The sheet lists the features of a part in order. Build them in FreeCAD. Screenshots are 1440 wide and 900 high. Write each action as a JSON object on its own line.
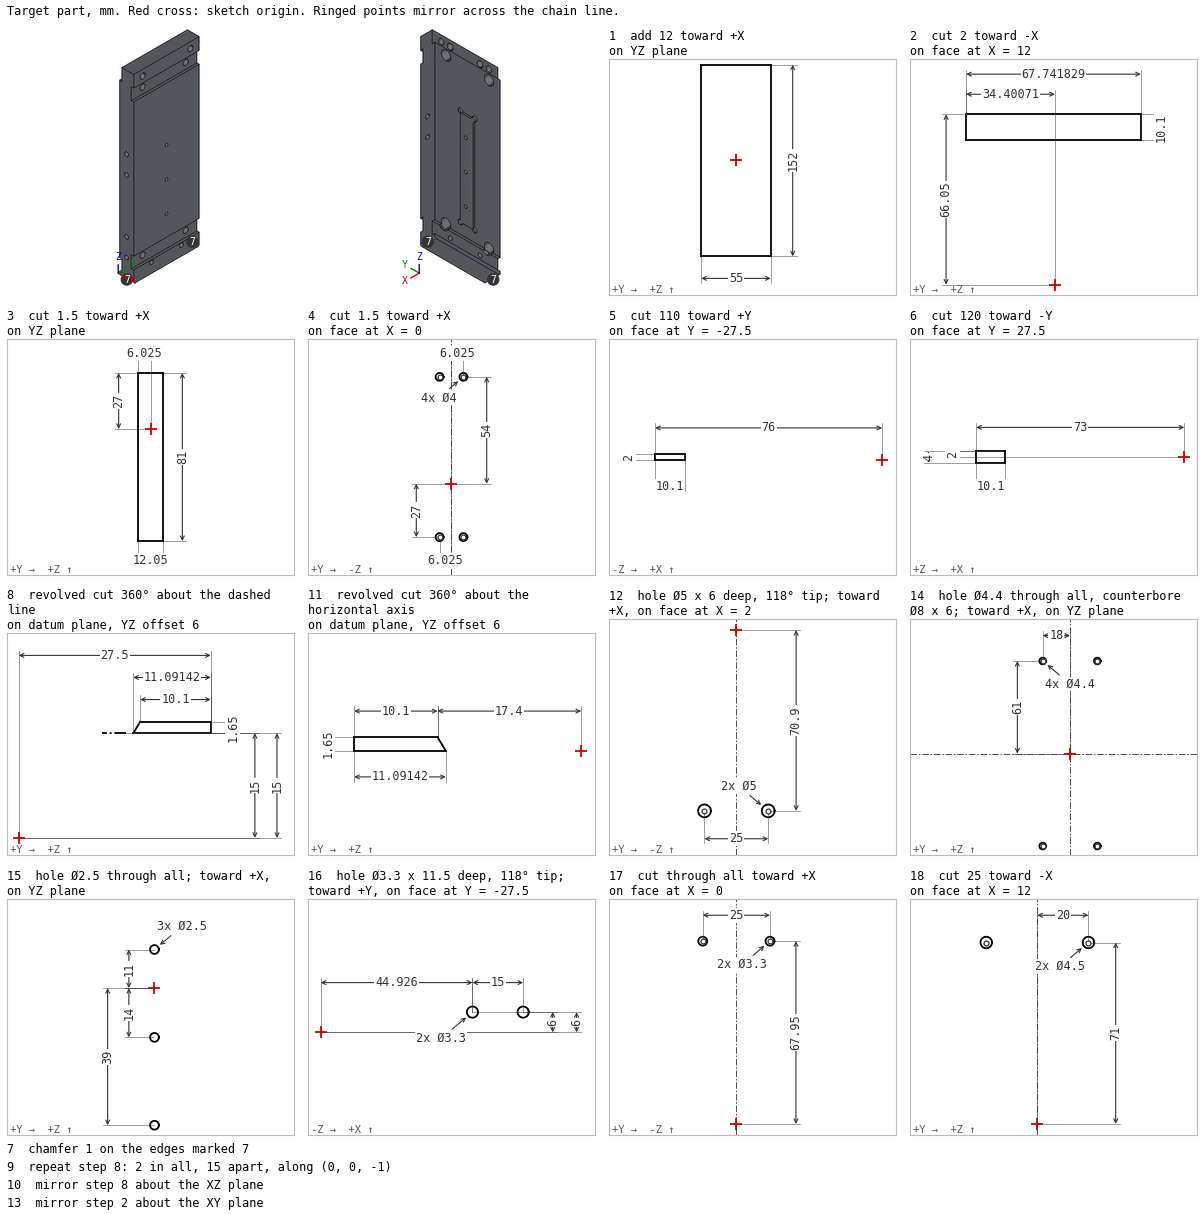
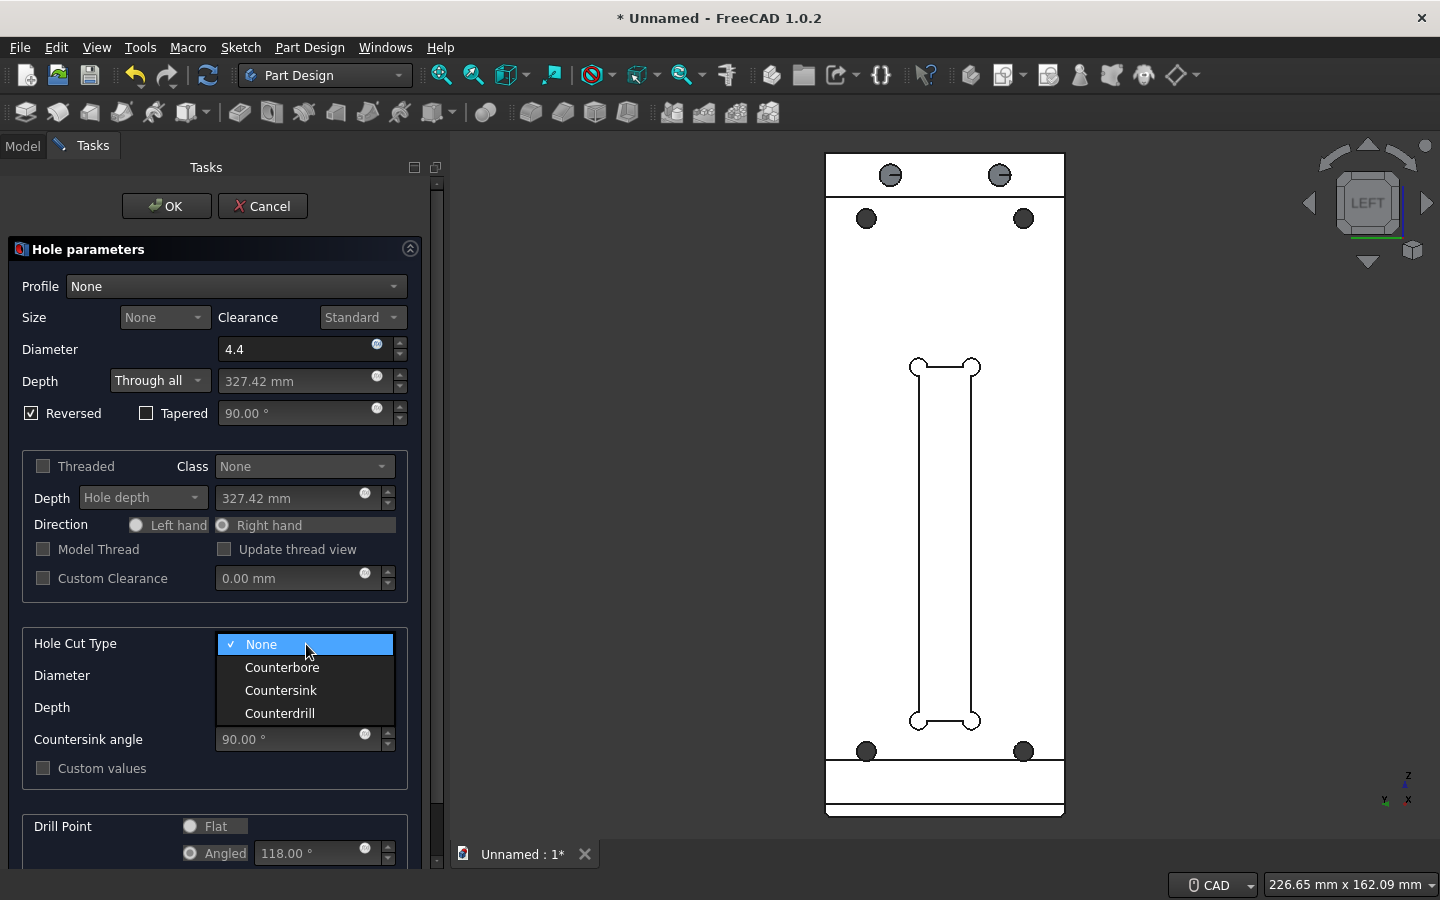
{"action": "left_click", "coordinate": [304, 668]}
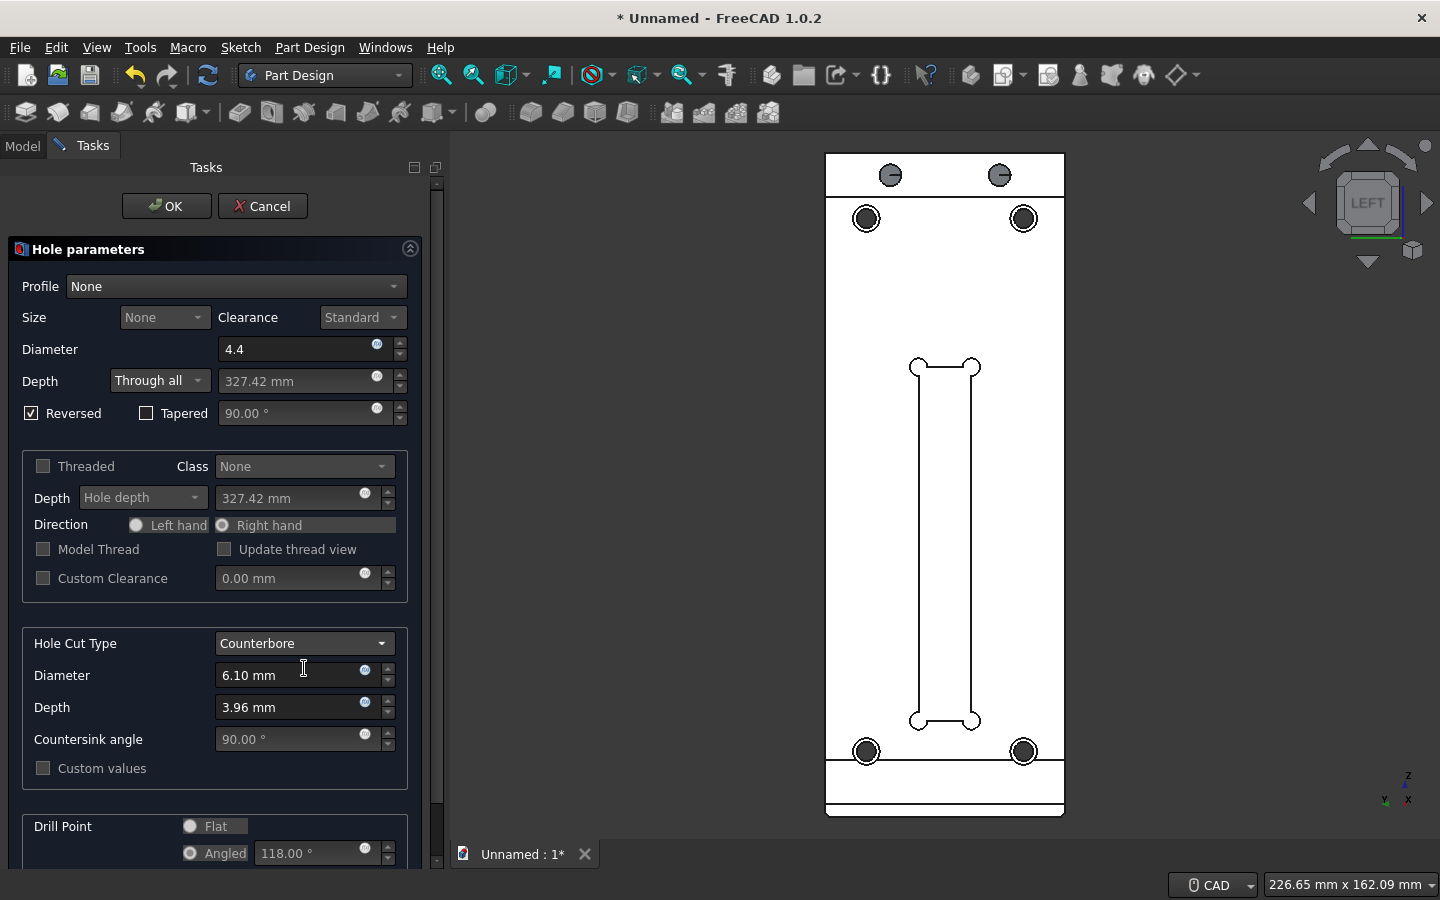
{"action": "triple_click", "coordinate": [298, 675]}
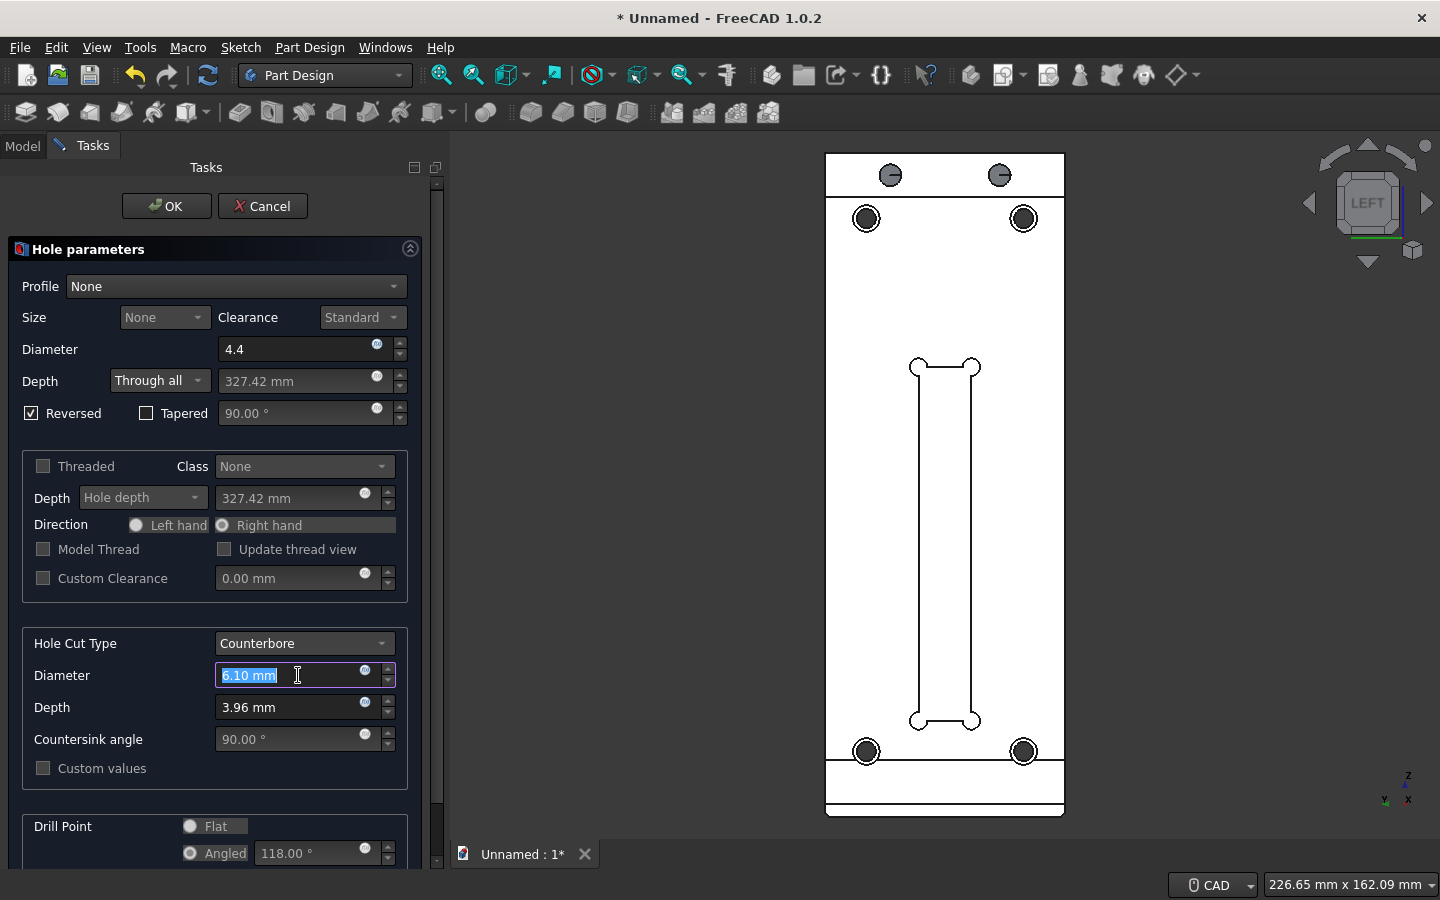
{"action": "type", "text": "8"}
{"action": "key", "text": "Tab"}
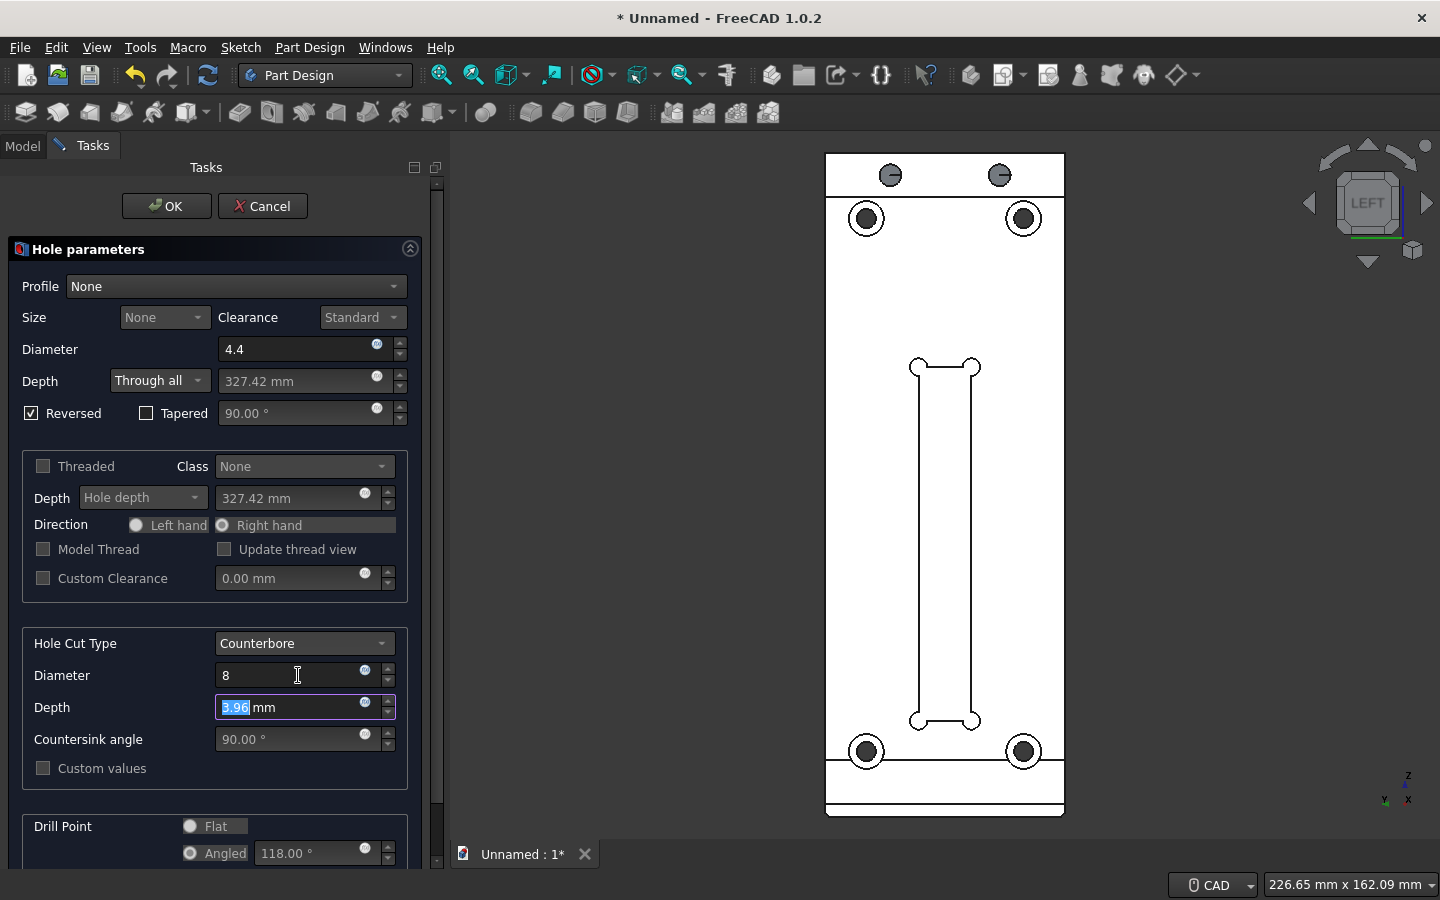
{"action": "type", "text": "6"}
{"action": "key", "text": "Tab"}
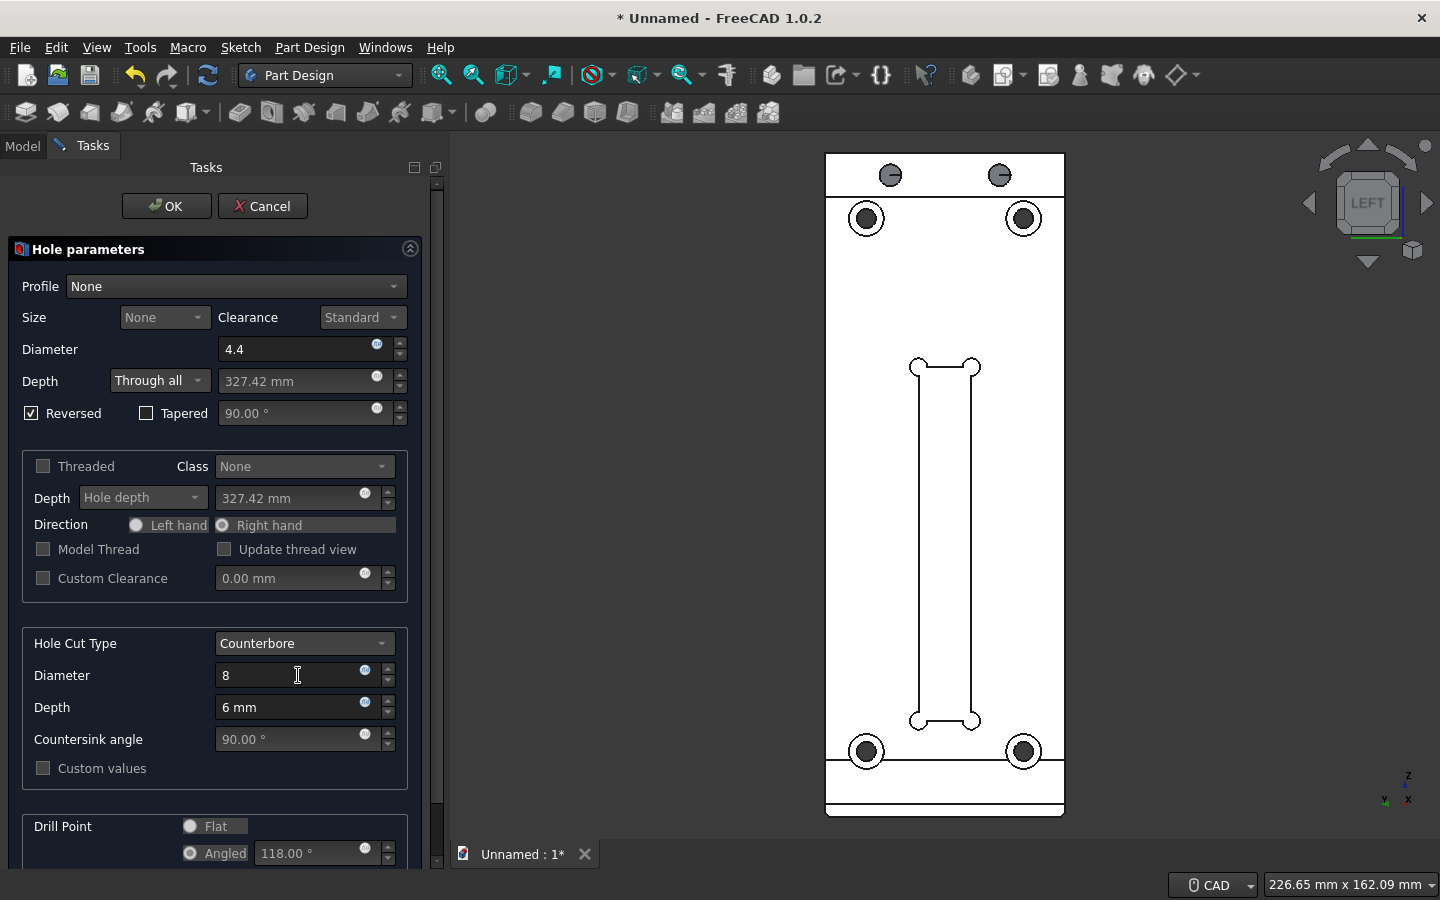
{"action": "left_click", "coordinate": [167, 206]}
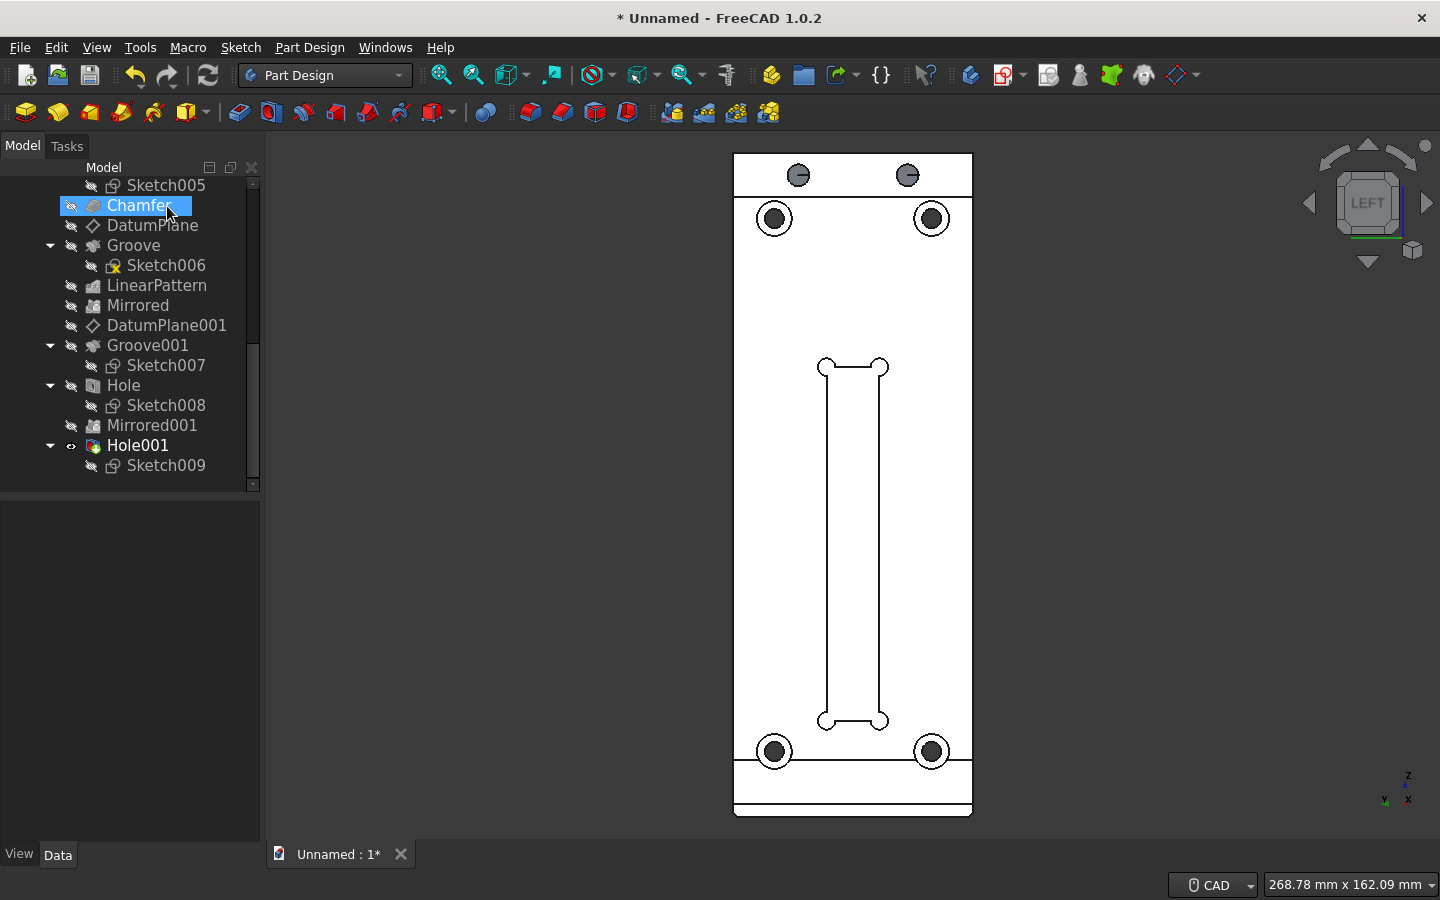
{"action": "left_click", "coordinate": [1004, 76]}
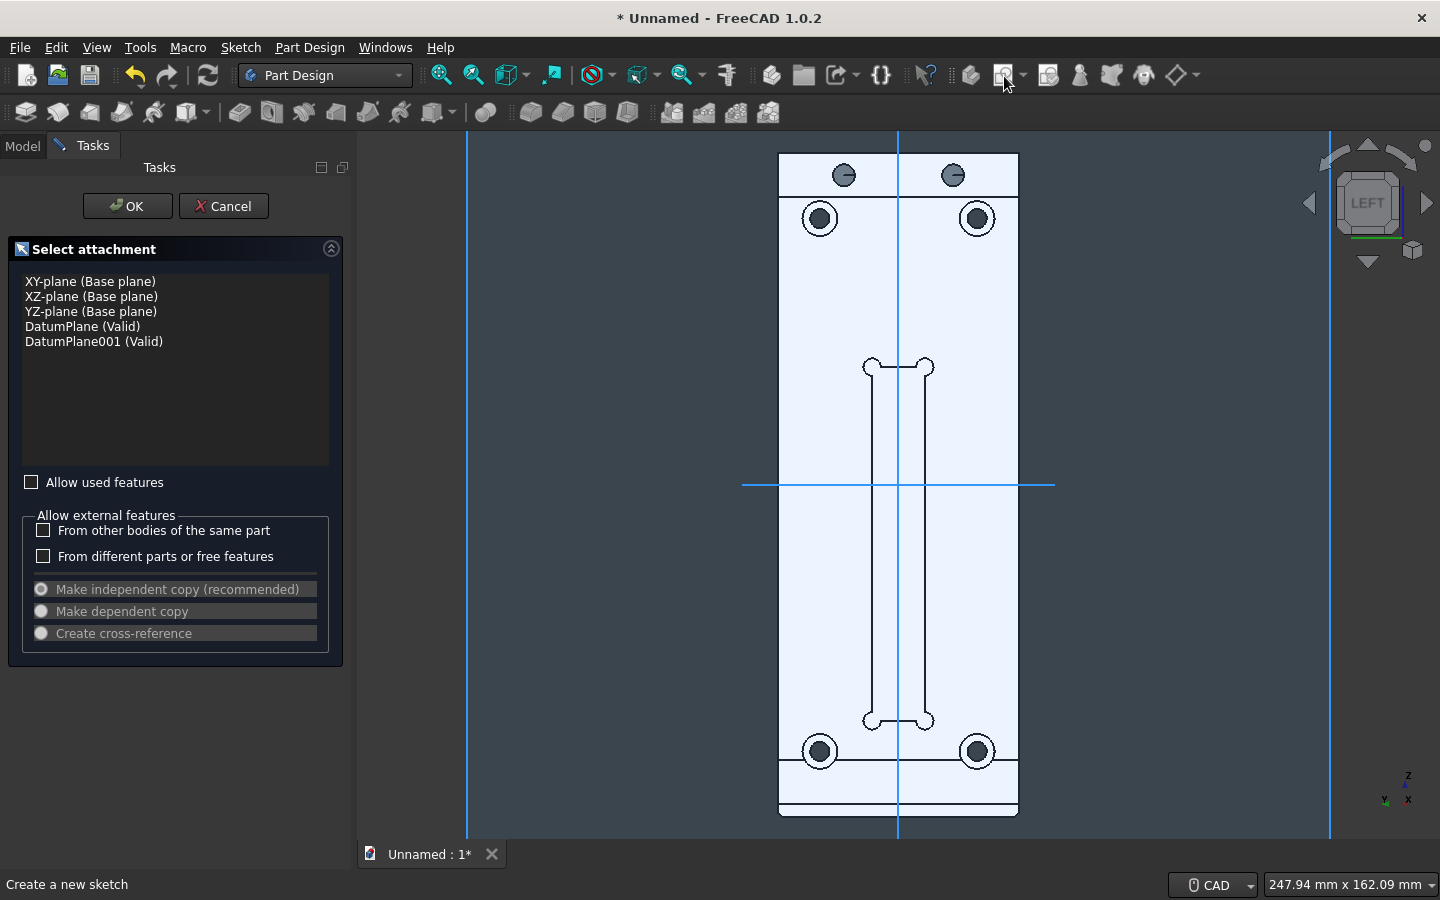
{"action": "left_click", "coordinate": [82, 312]}